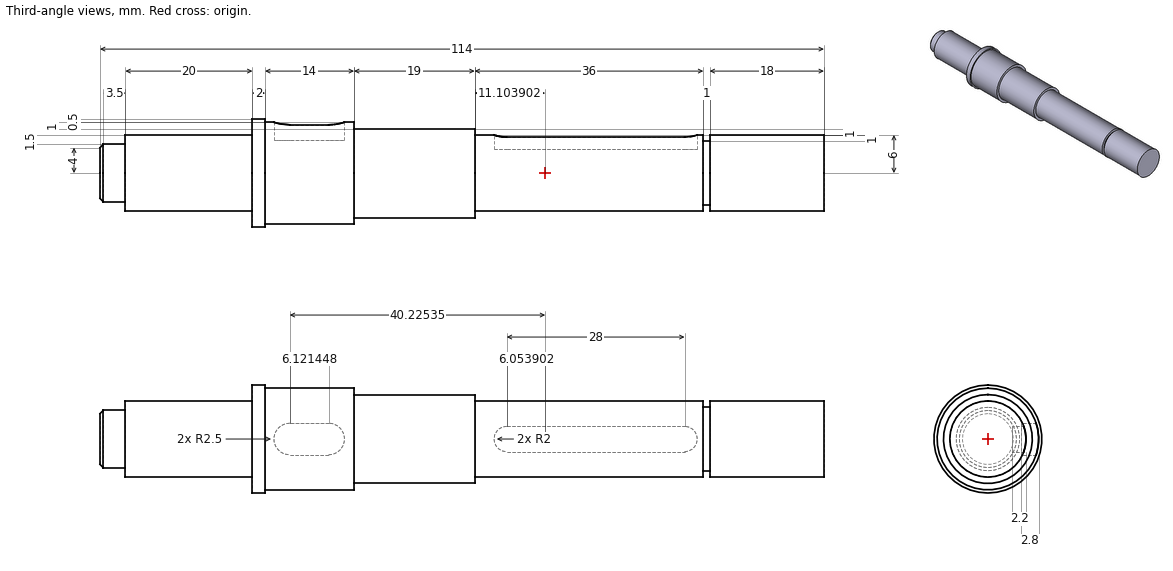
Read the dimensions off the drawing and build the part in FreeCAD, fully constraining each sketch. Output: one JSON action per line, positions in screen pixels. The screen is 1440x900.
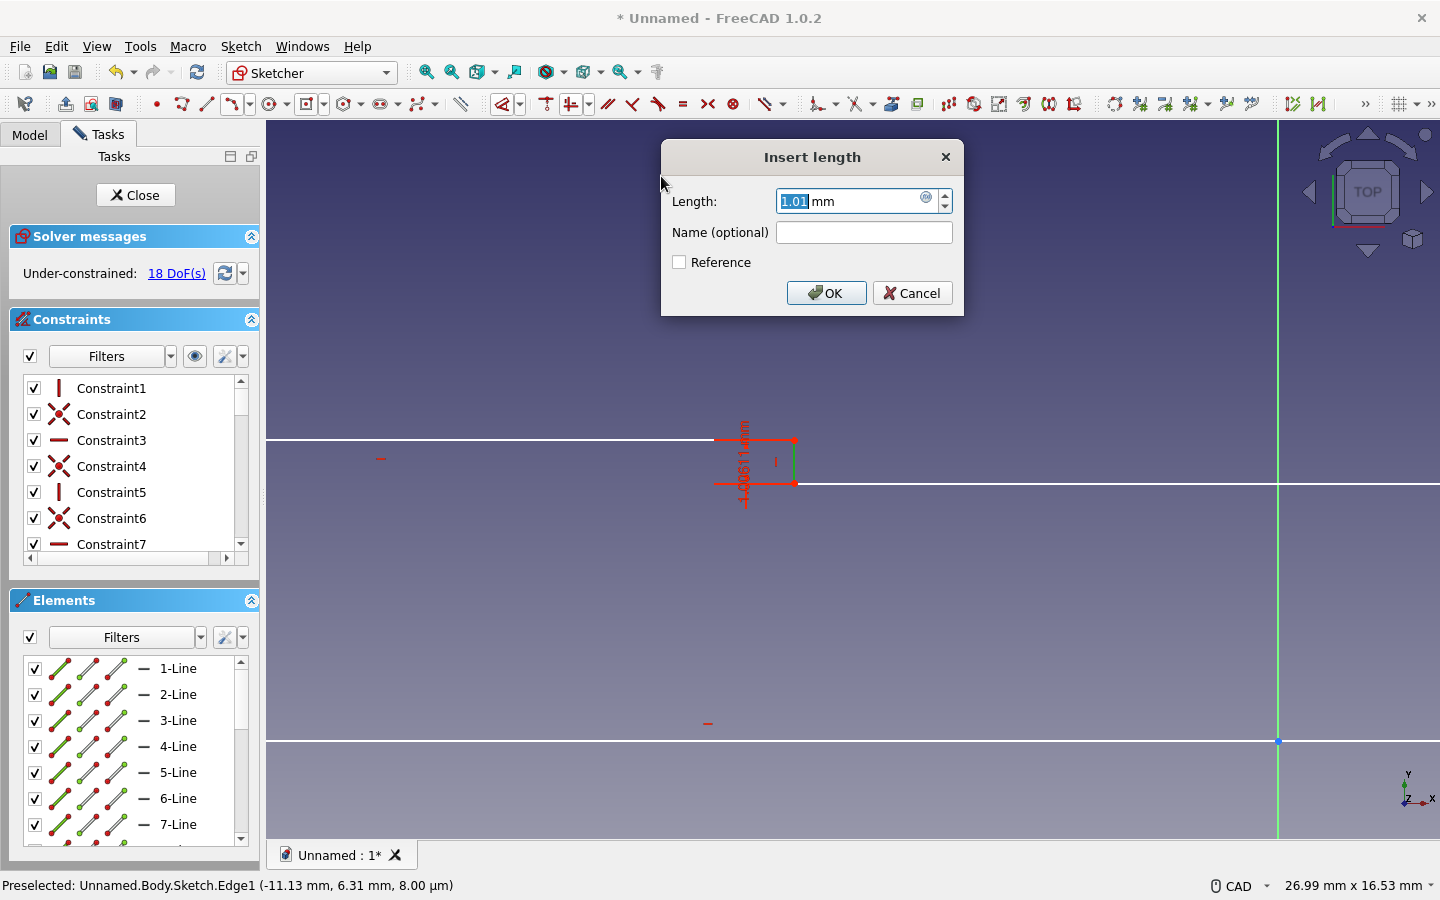
{"action": "type", "text": "1"}
{"action": "key", "text": "Return"}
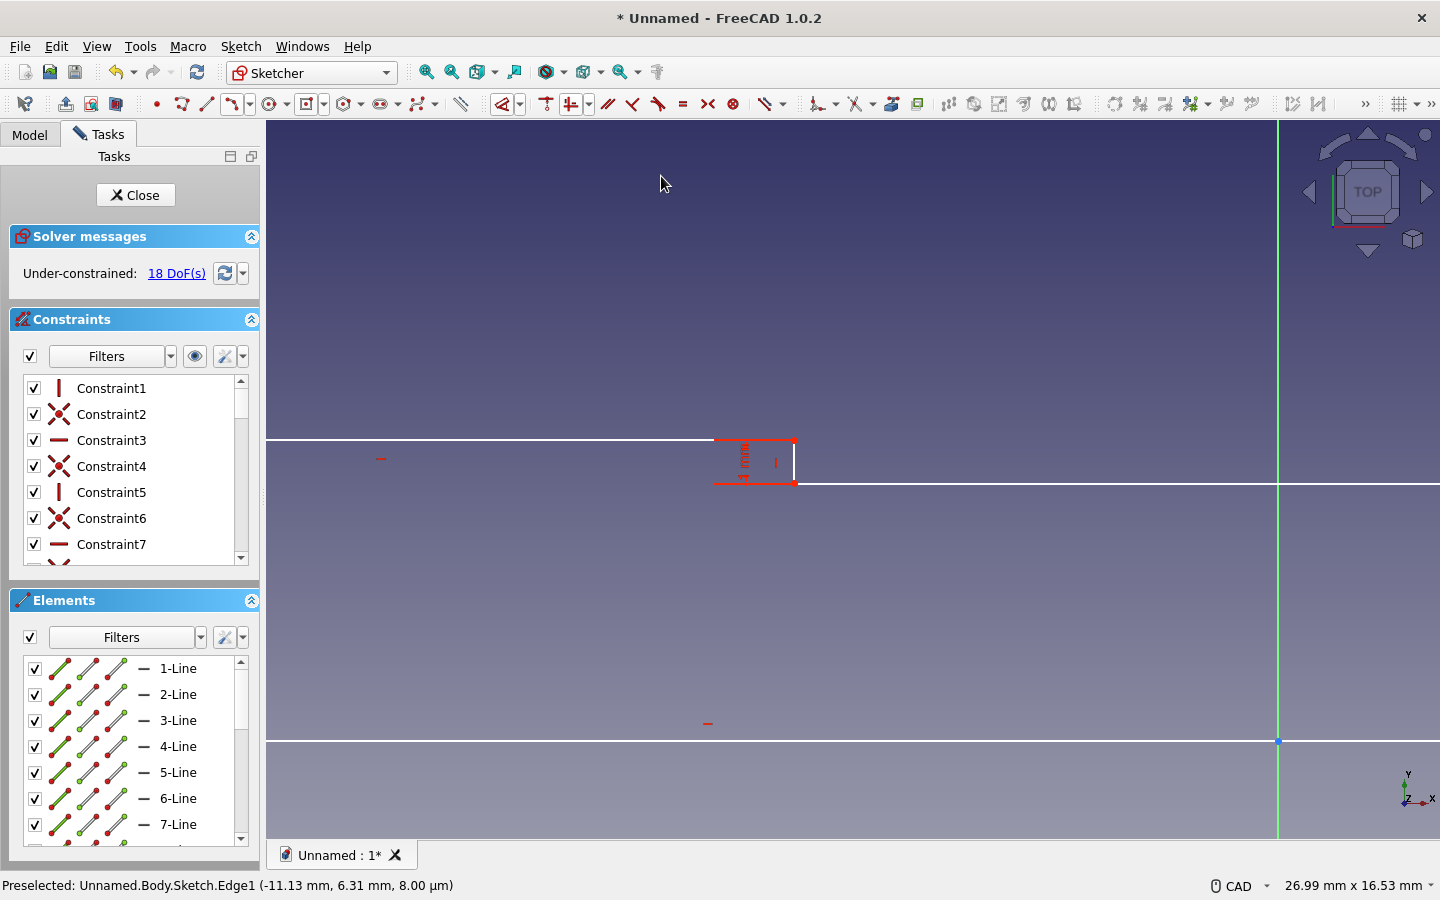
{"action": "scroll", "coordinate": [796, 467], "scroll_direction": "down", "scroll_amount": 10}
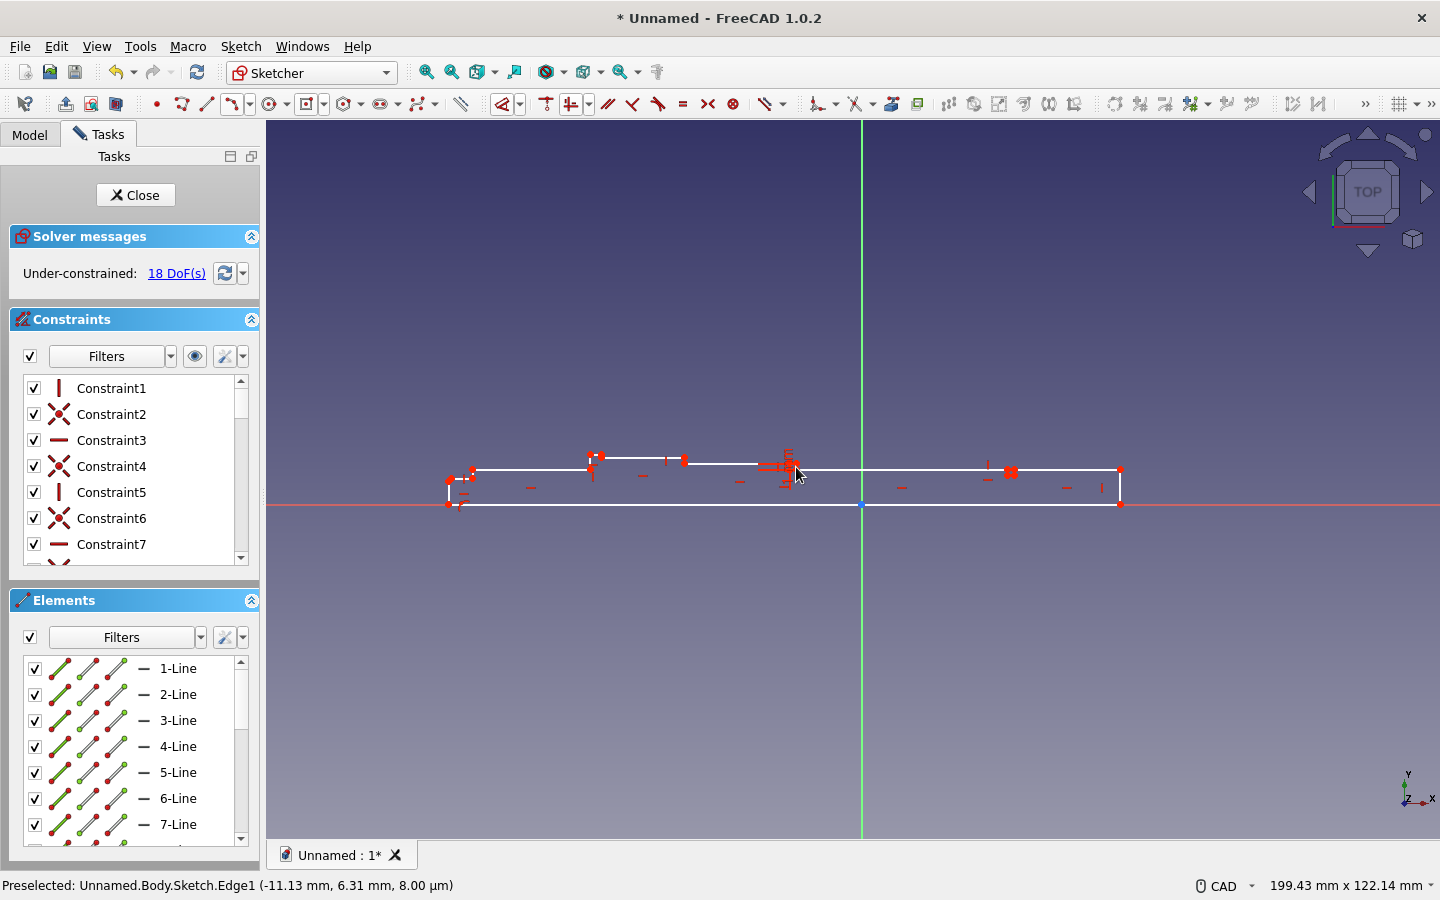
{"action": "scroll", "coordinate": [684, 462], "scroll_direction": "up", "scroll_amount": 11}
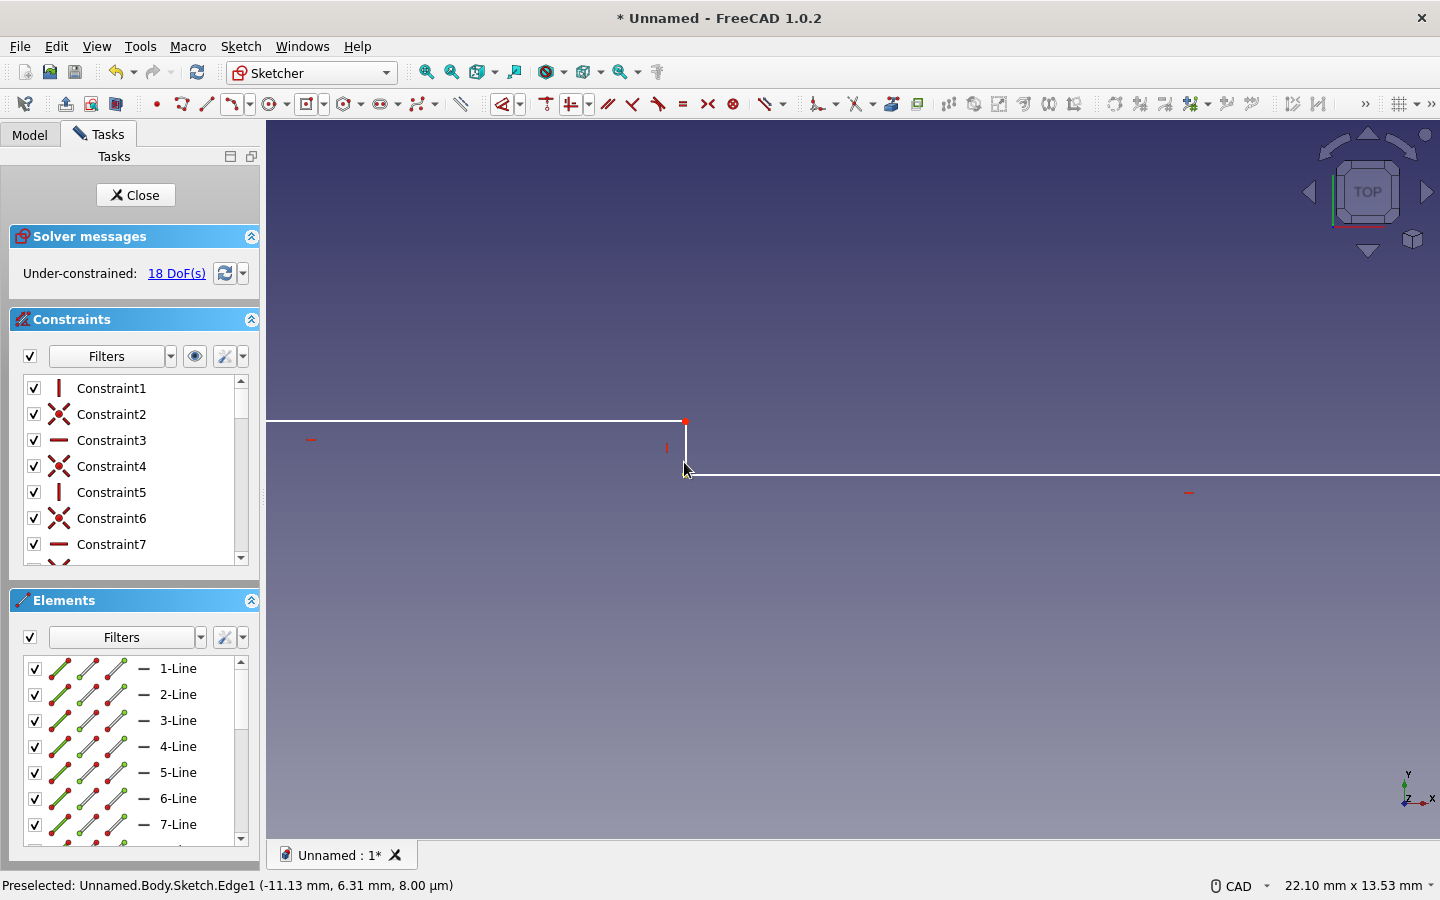
{"action": "left_click", "coordinate": [686, 458]}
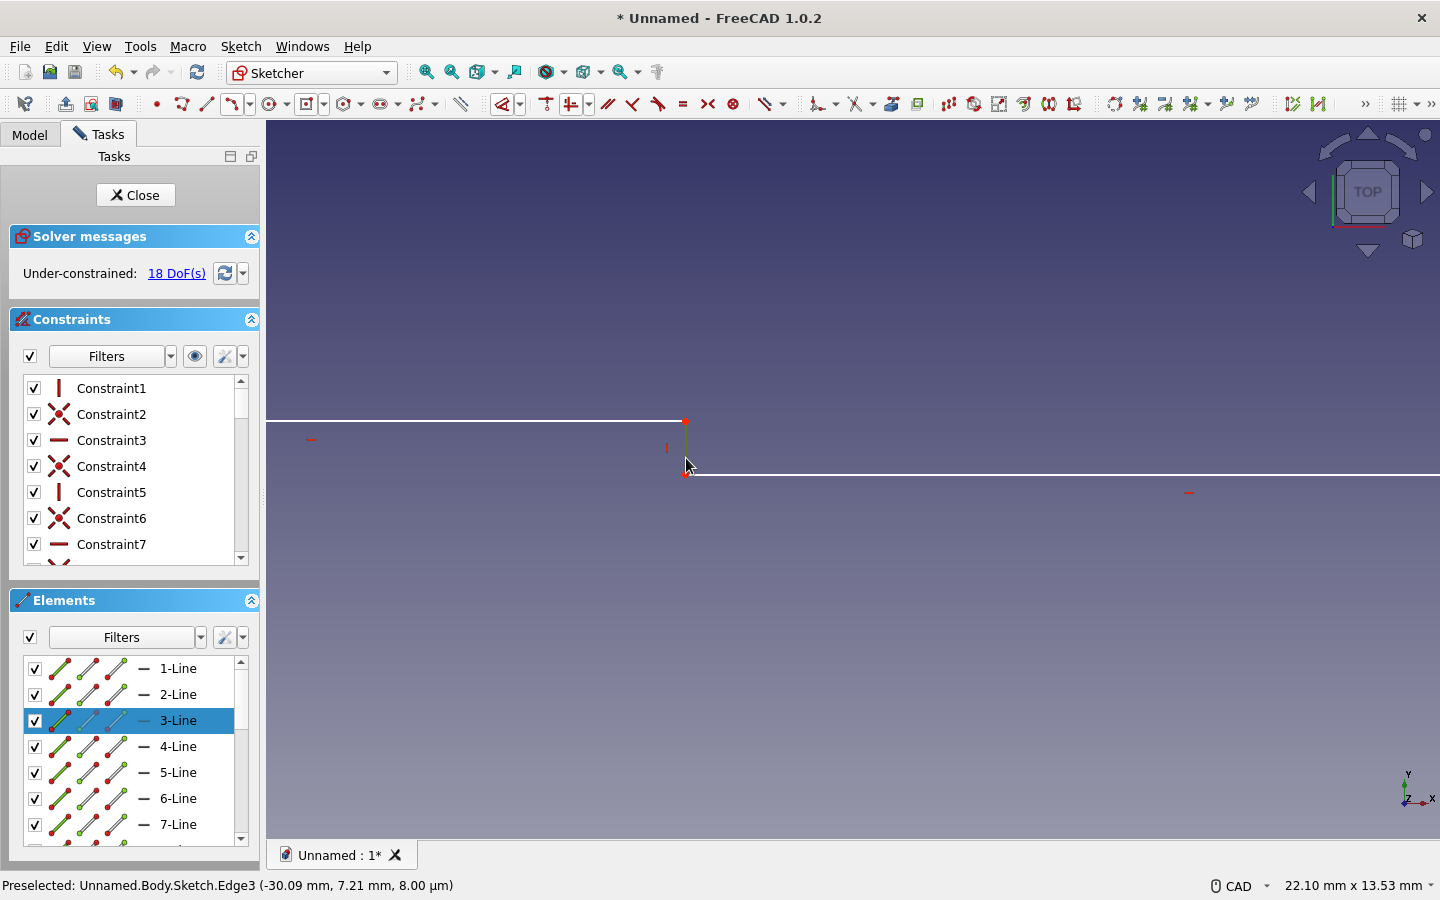
{"action": "key", "text": "i"}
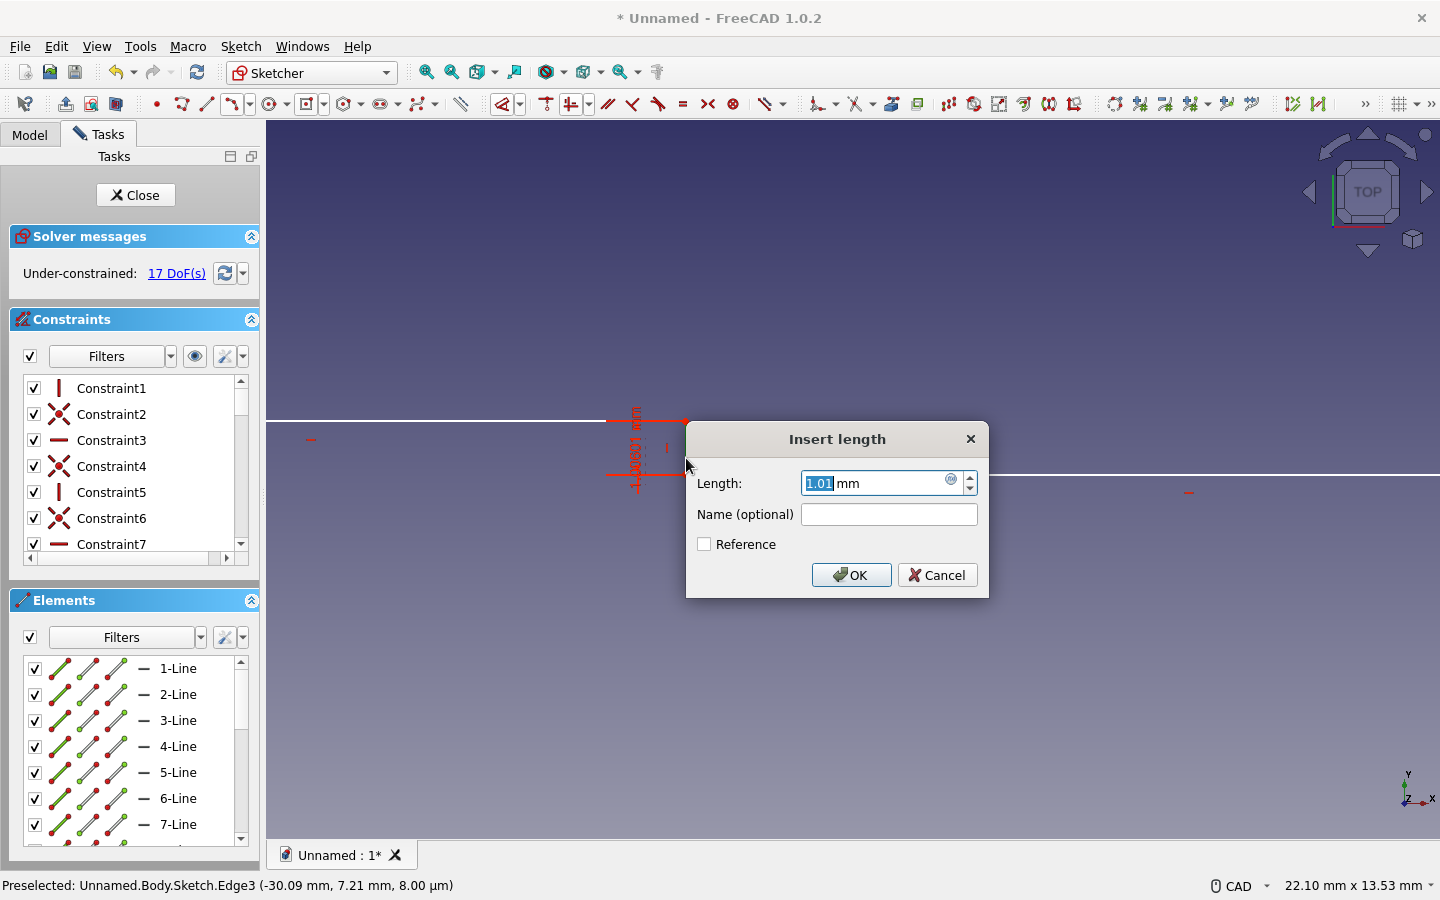
{"action": "type", "text": "1"}
{"action": "key", "text": "Return"}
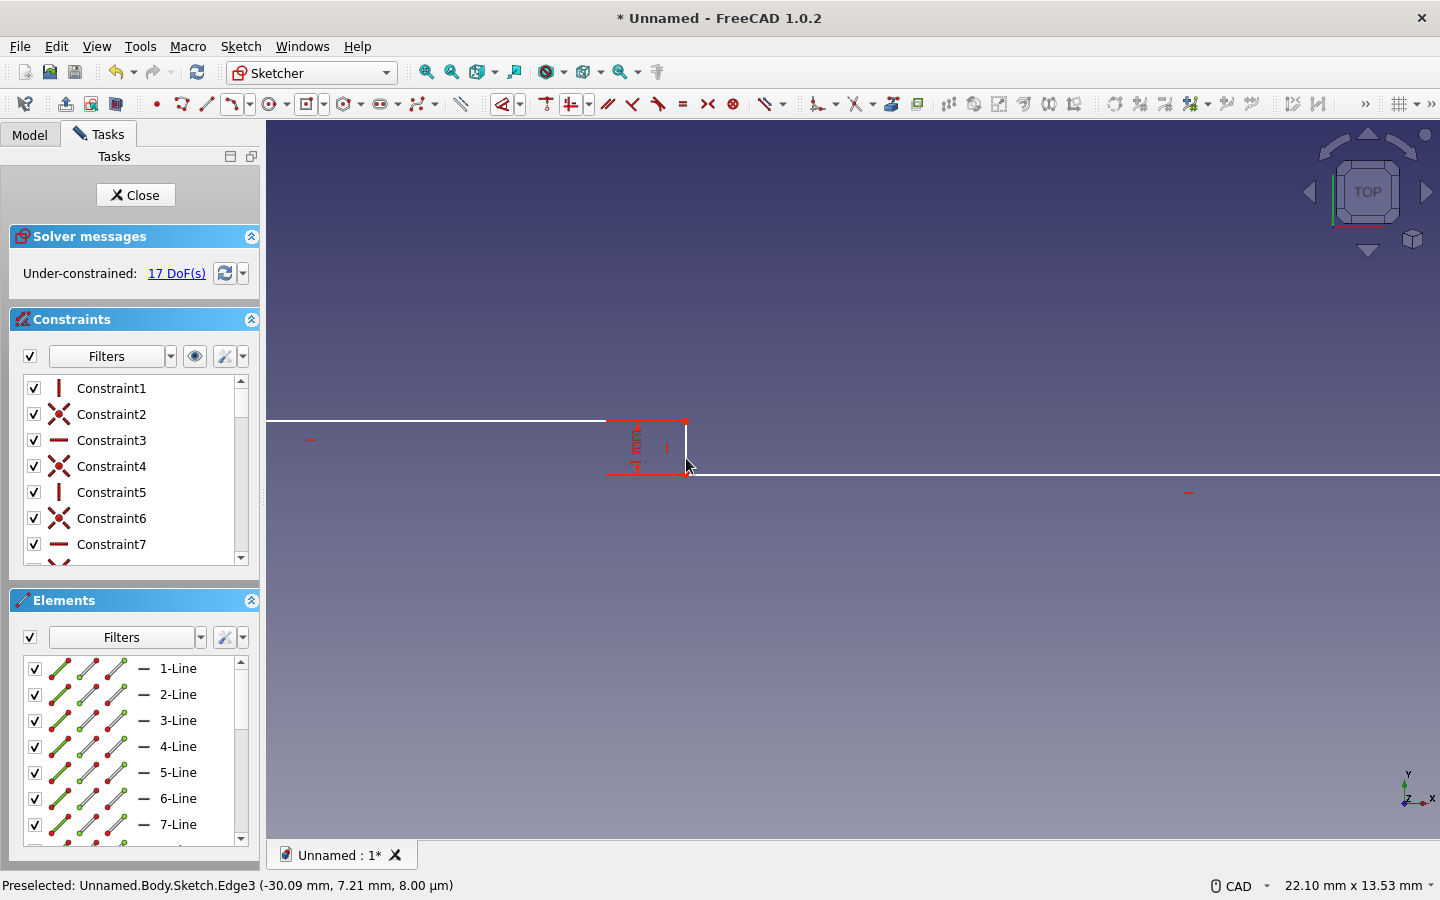
{"action": "scroll", "coordinate": [684, 462], "scroll_direction": "down", "scroll_amount": 11}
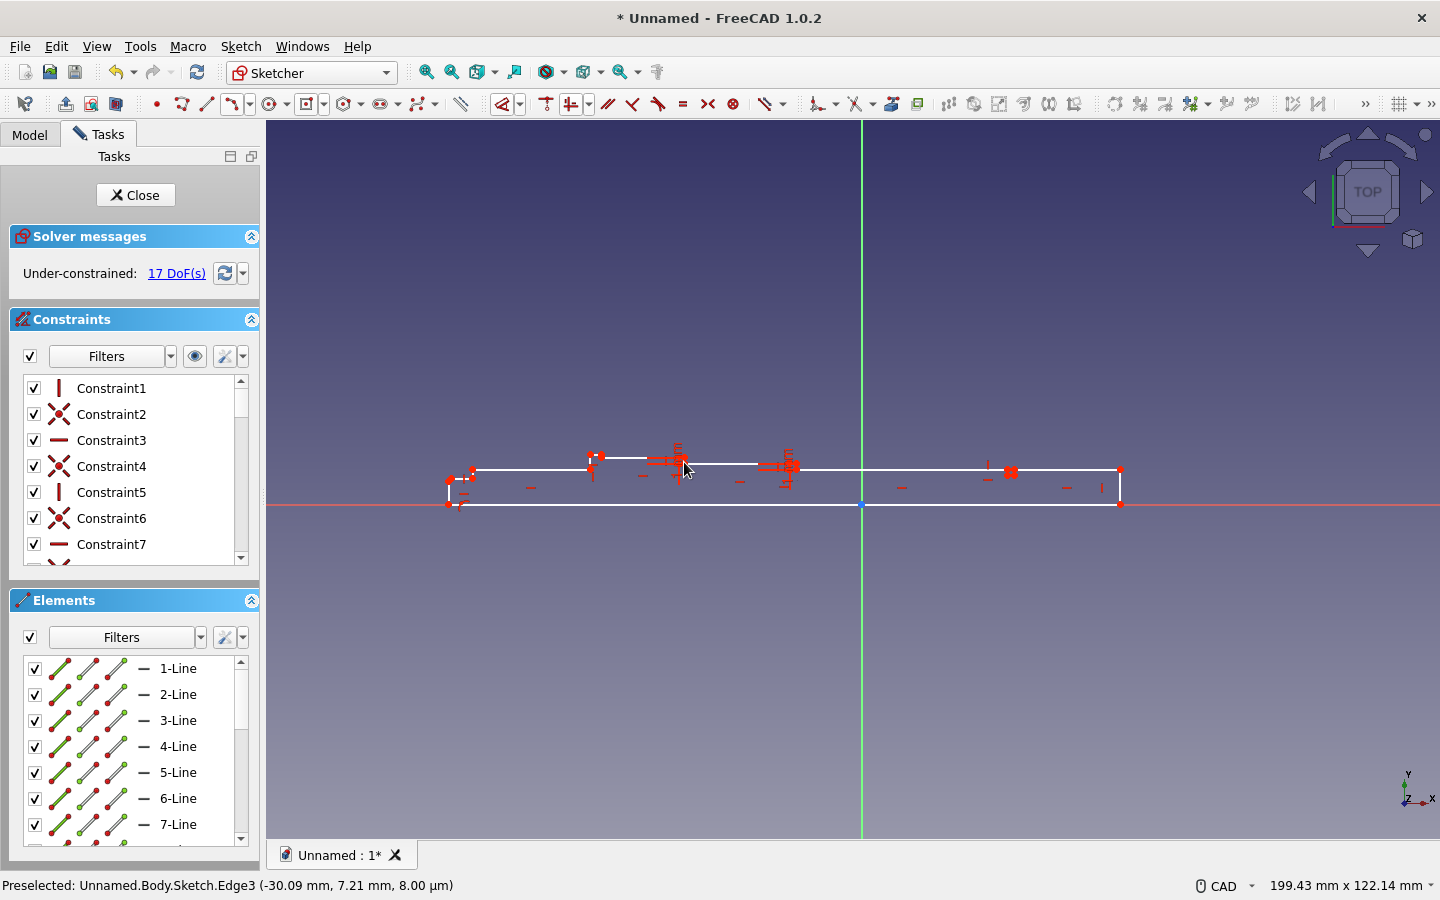
{"action": "scroll", "coordinate": [598, 455], "scroll_direction": "up", "scroll_amount": 7}